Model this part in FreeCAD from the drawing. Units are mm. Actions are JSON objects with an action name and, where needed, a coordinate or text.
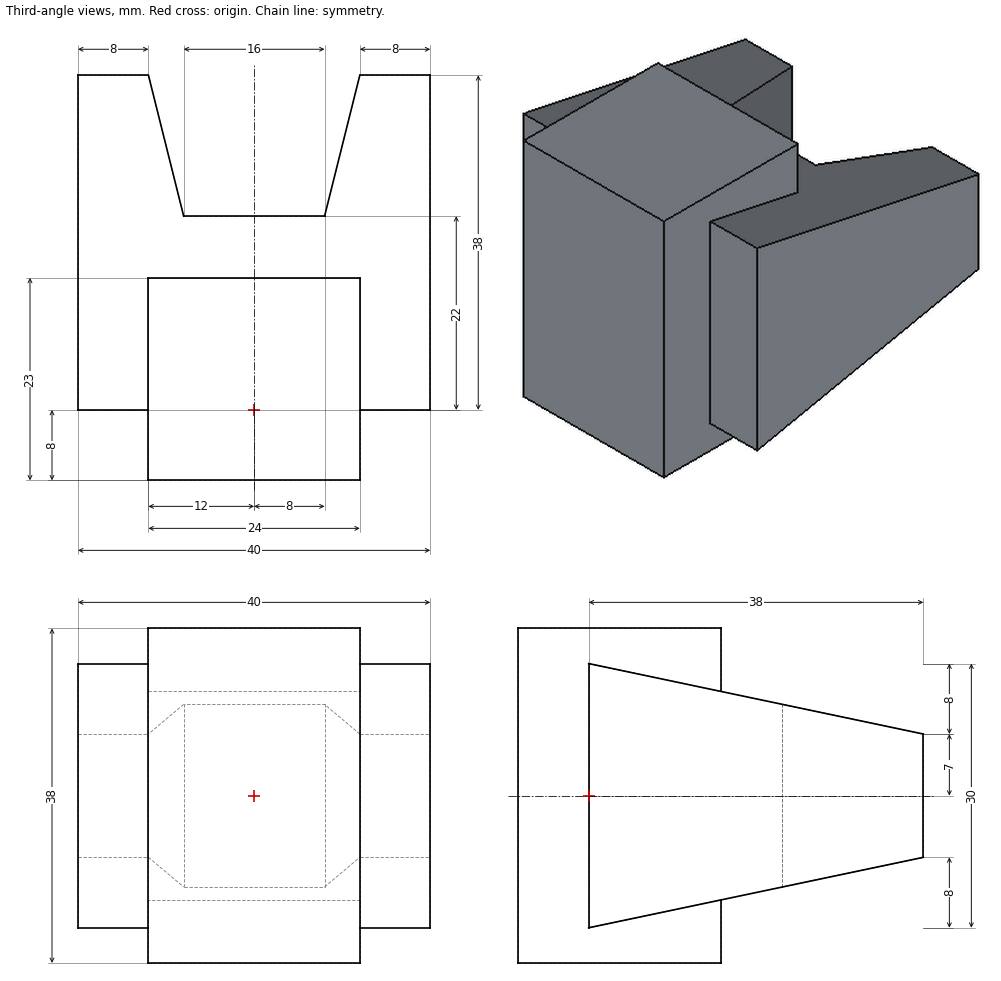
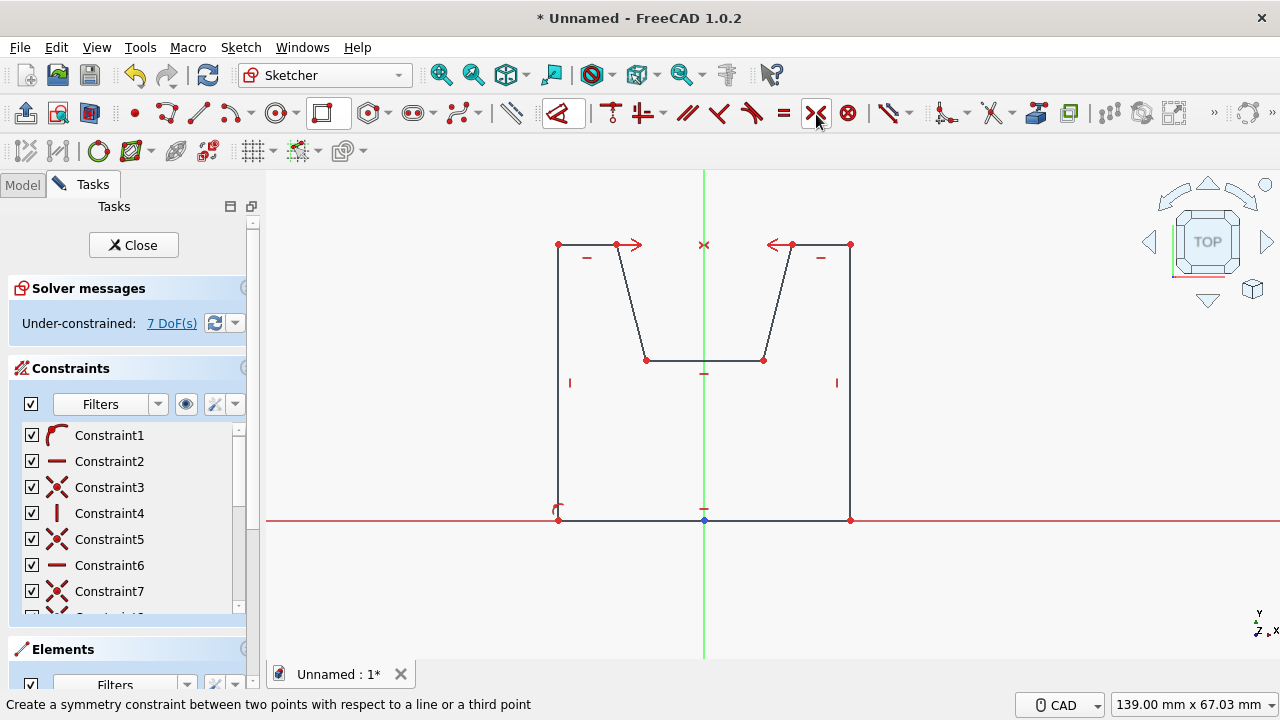
{"action": "left_click", "coordinate": [558, 114]}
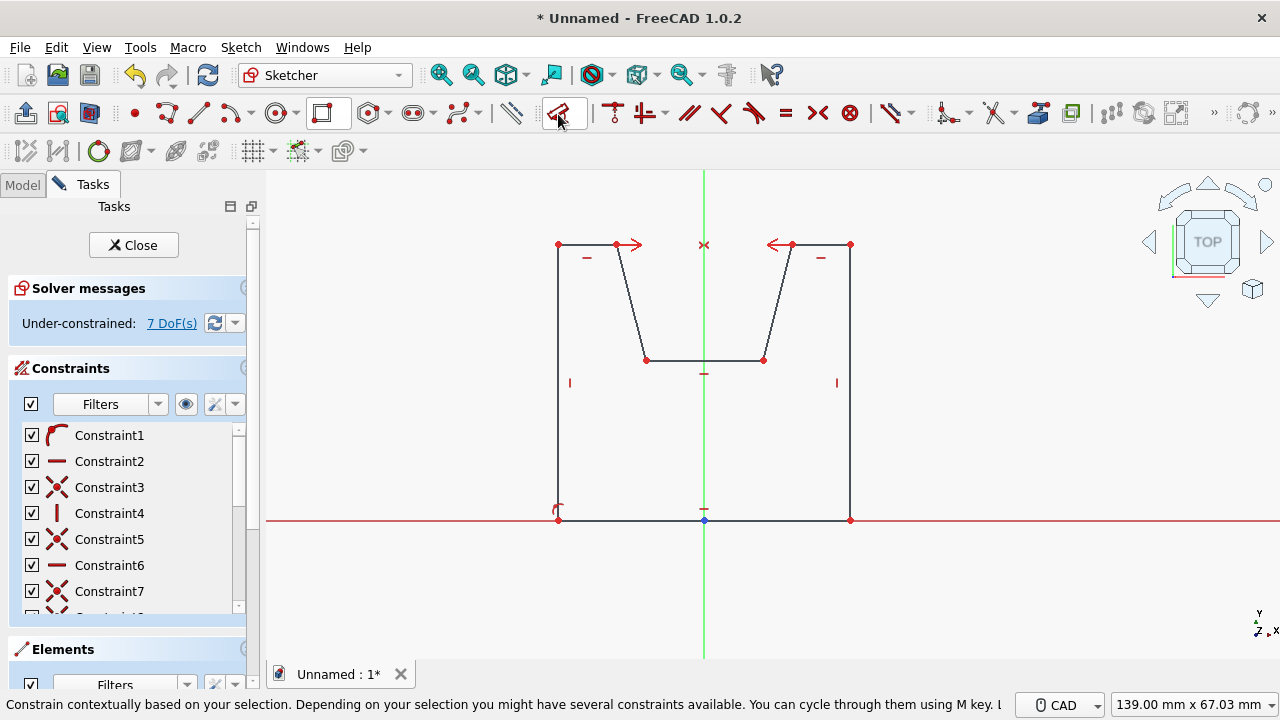
{"action": "left_click", "coordinate": [833, 245]}
{"action": "left_click", "coordinate": [821, 211]}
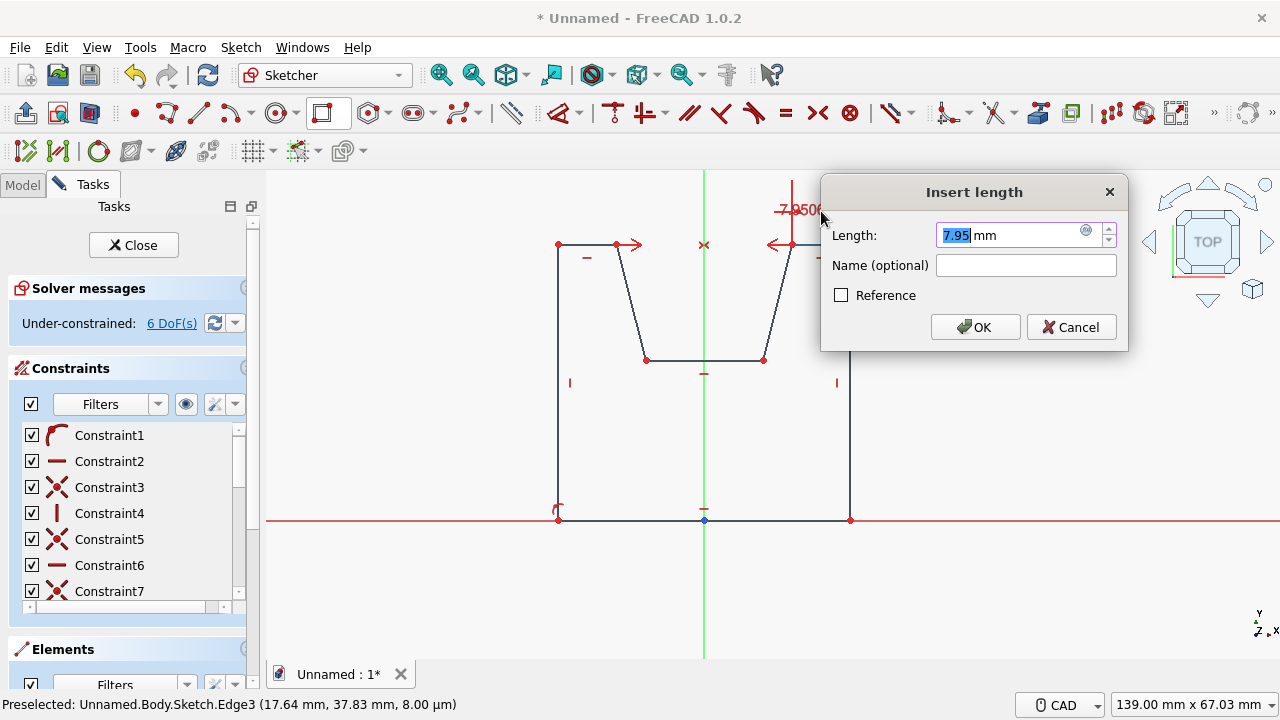
{"action": "type", "text": "8"}
{"action": "key", "text": "Return"}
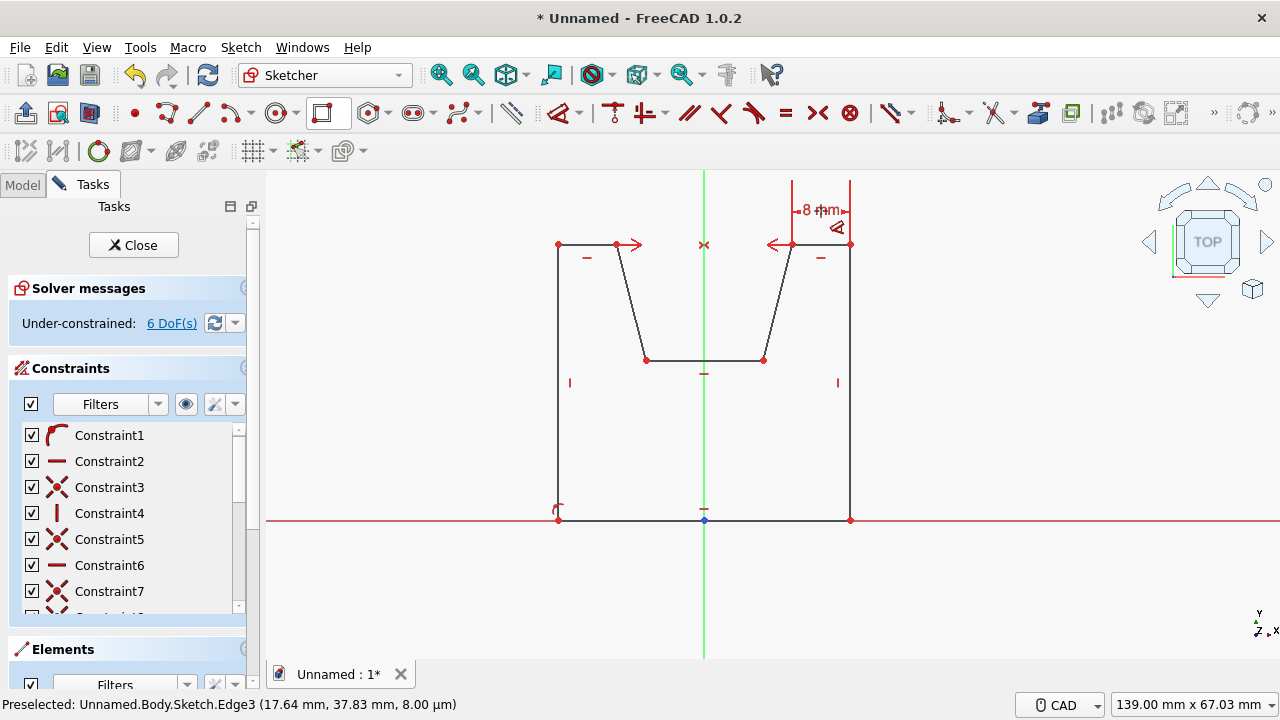
{"action": "left_click", "coordinate": [599, 245]}
{"action": "left_click", "coordinate": [587, 211]}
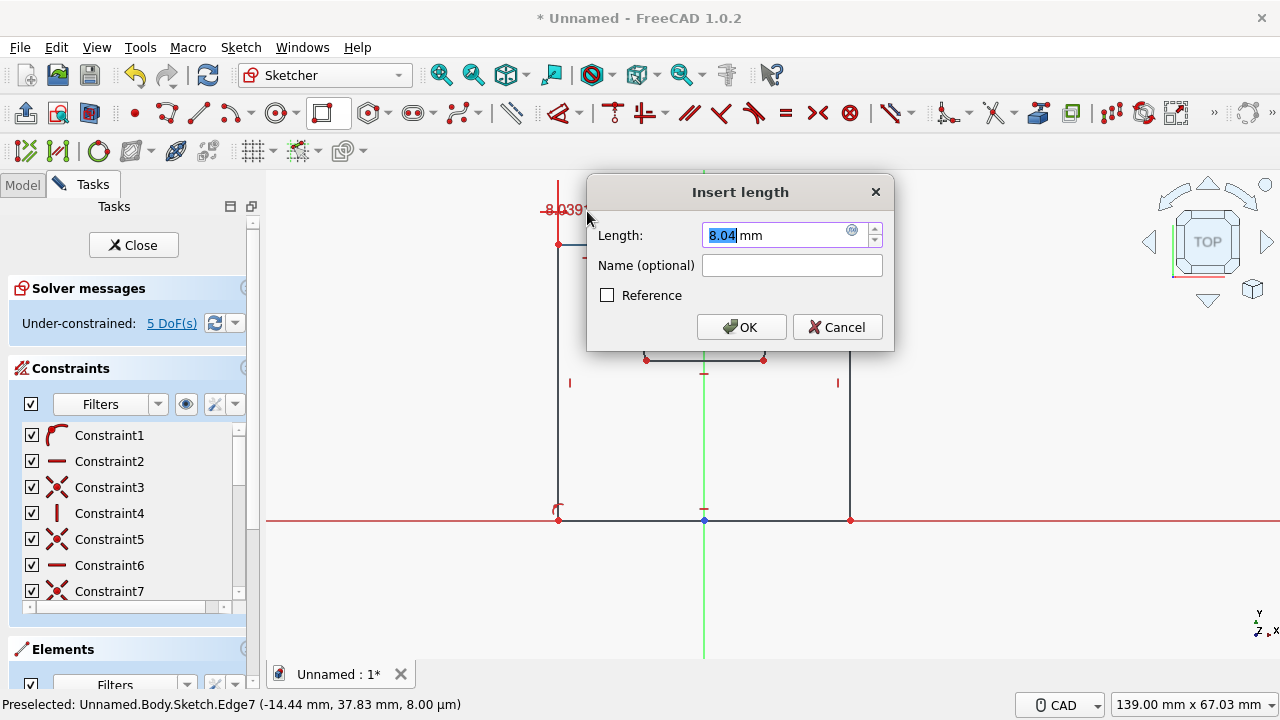
{"action": "type", "text": "8"}
{"action": "key", "text": "Return"}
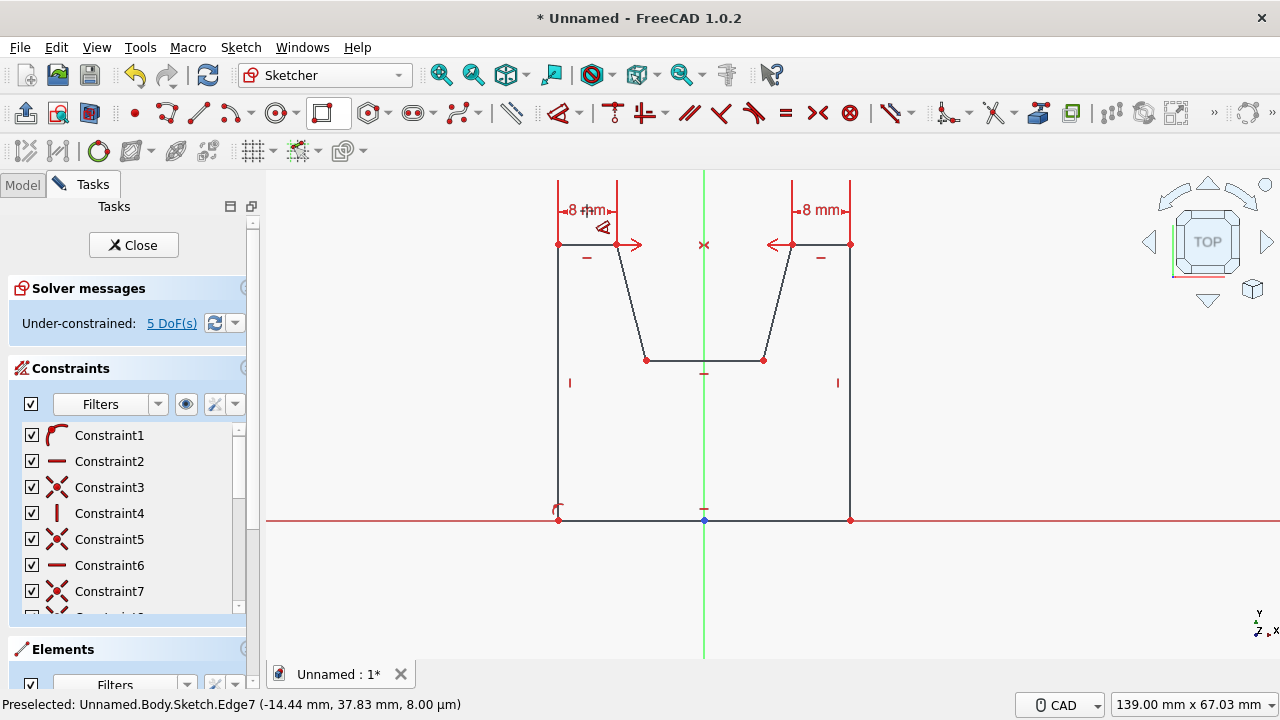
{"action": "left_click", "coordinate": [646, 521]}
{"action": "left_click", "coordinate": [637, 555]}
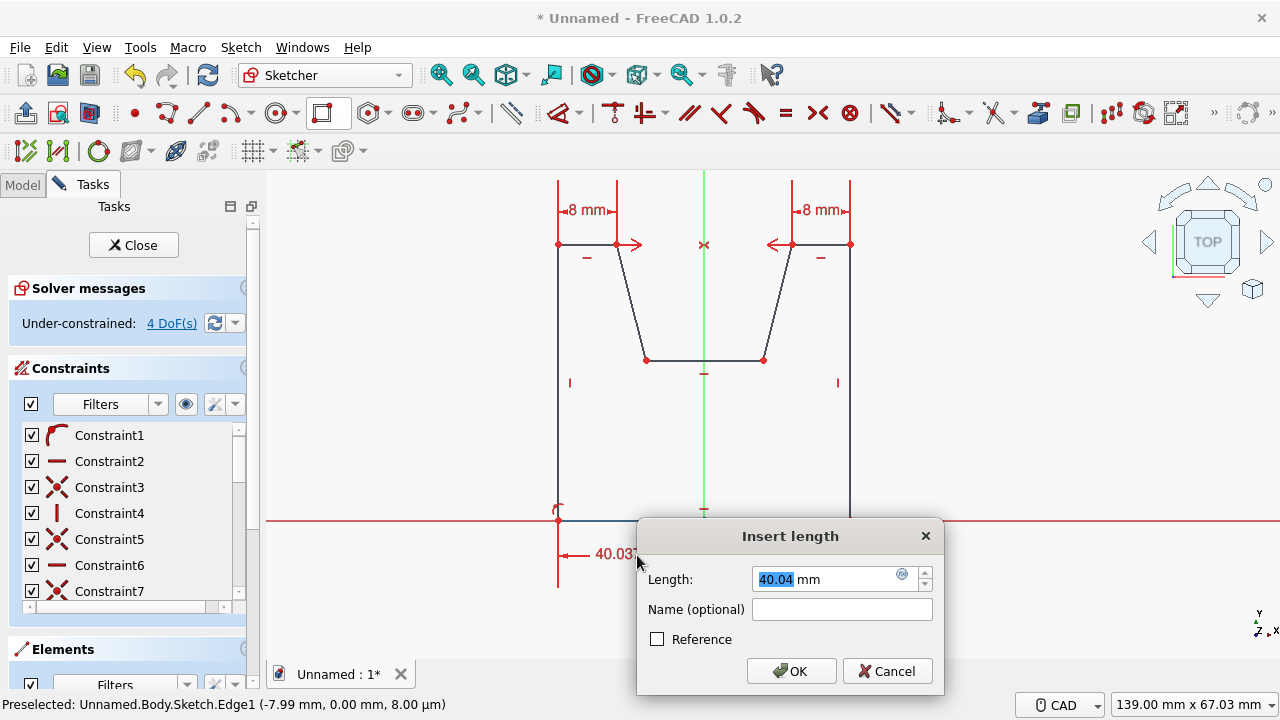
{"action": "type", "text": "40"}
{"action": "key", "text": "Return"}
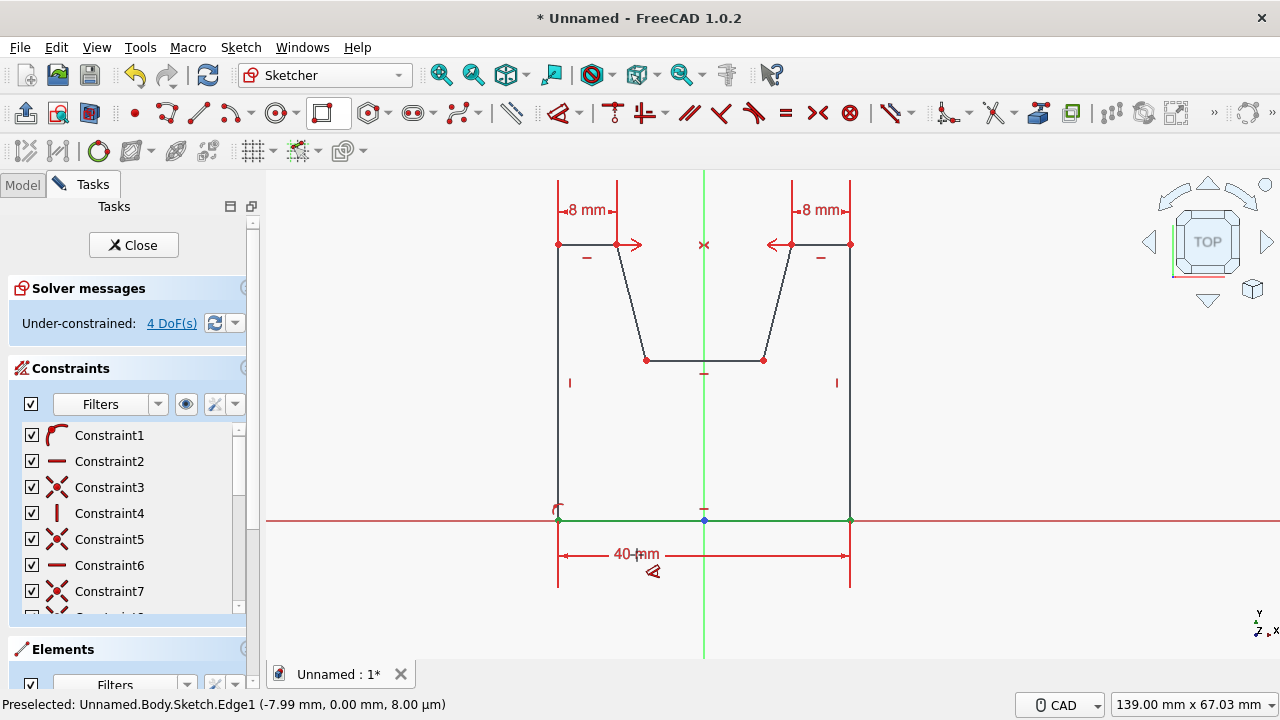
{"action": "left_click", "coordinate": [850, 438]}
{"action": "left_click", "coordinate": [884, 383]}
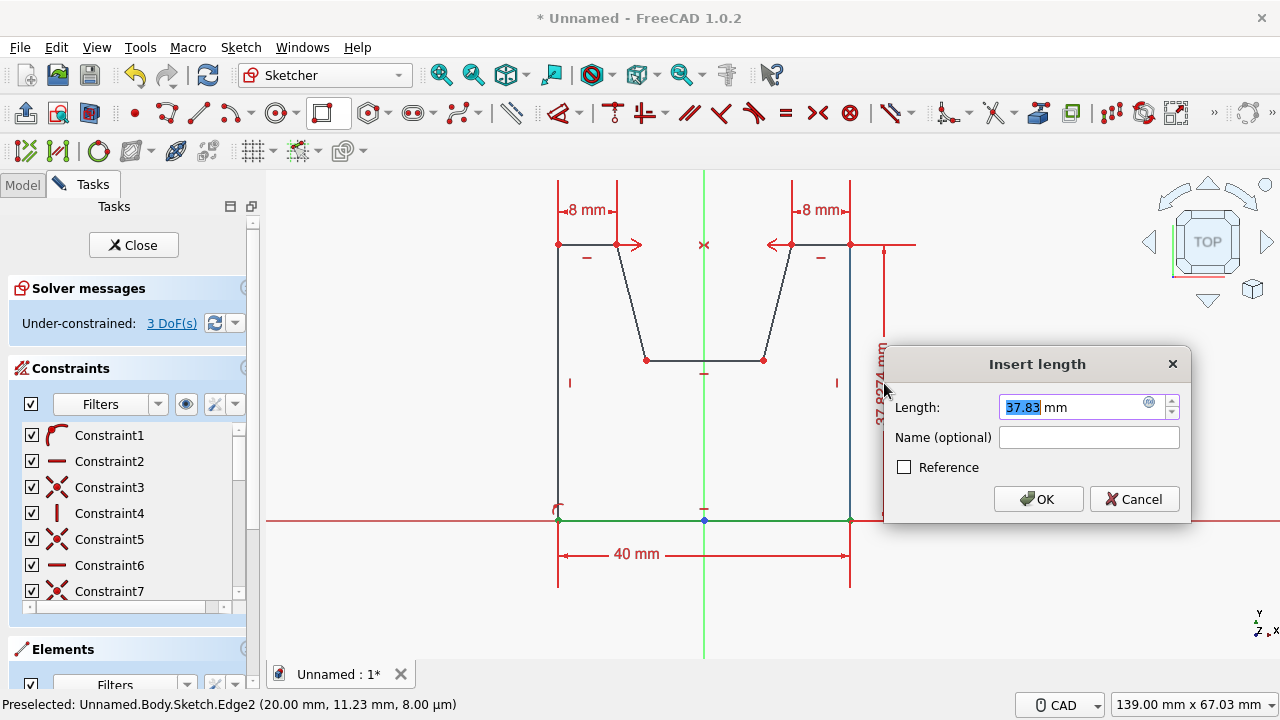
{"action": "type", "text": "38"}
{"action": "key", "text": "Return"}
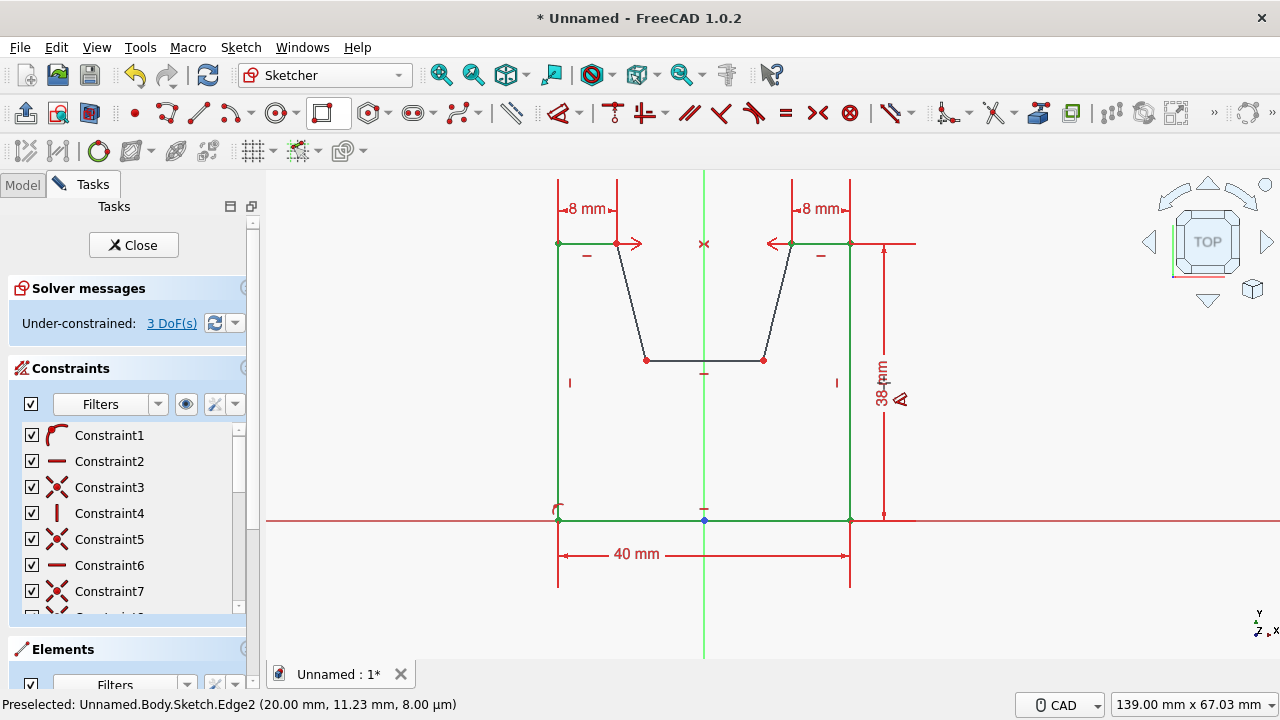
{"action": "left_click", "coordinate": [728, 361]}
{"action": "left_click", "coordinate": [678, 327]}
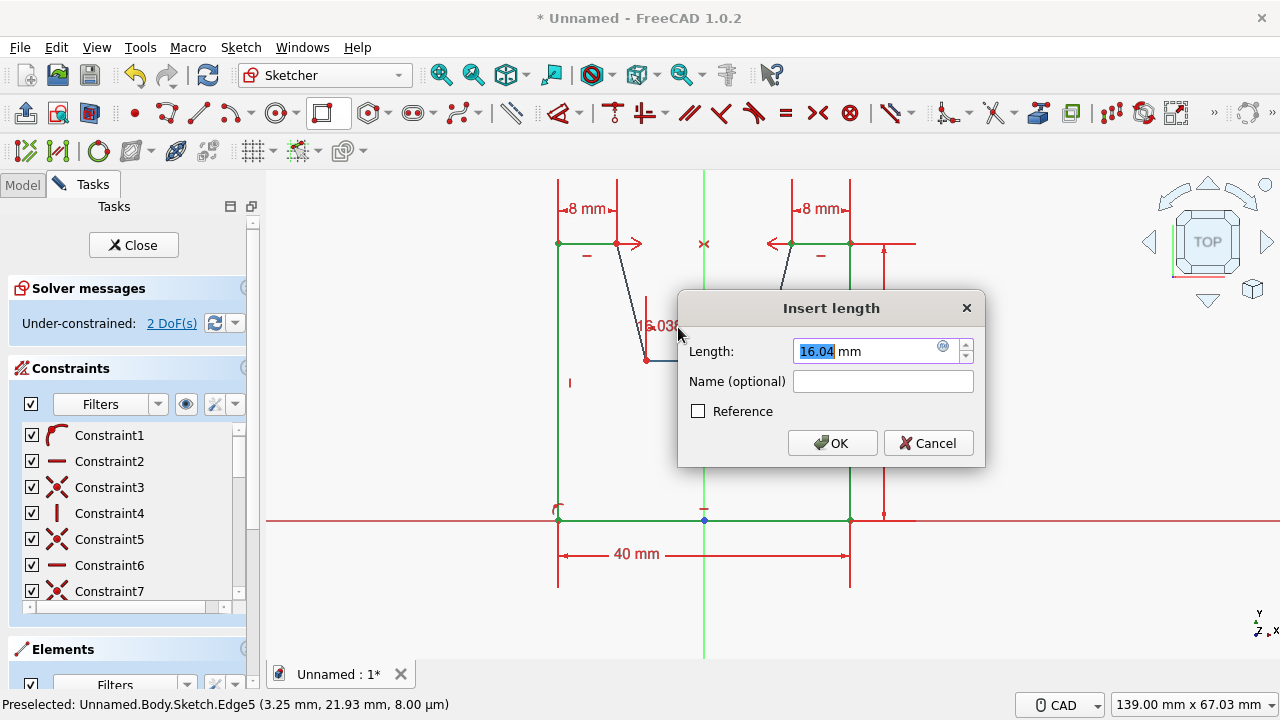
{"action": "type", "text": "16"}
{"action": "key", "text": "Return"}